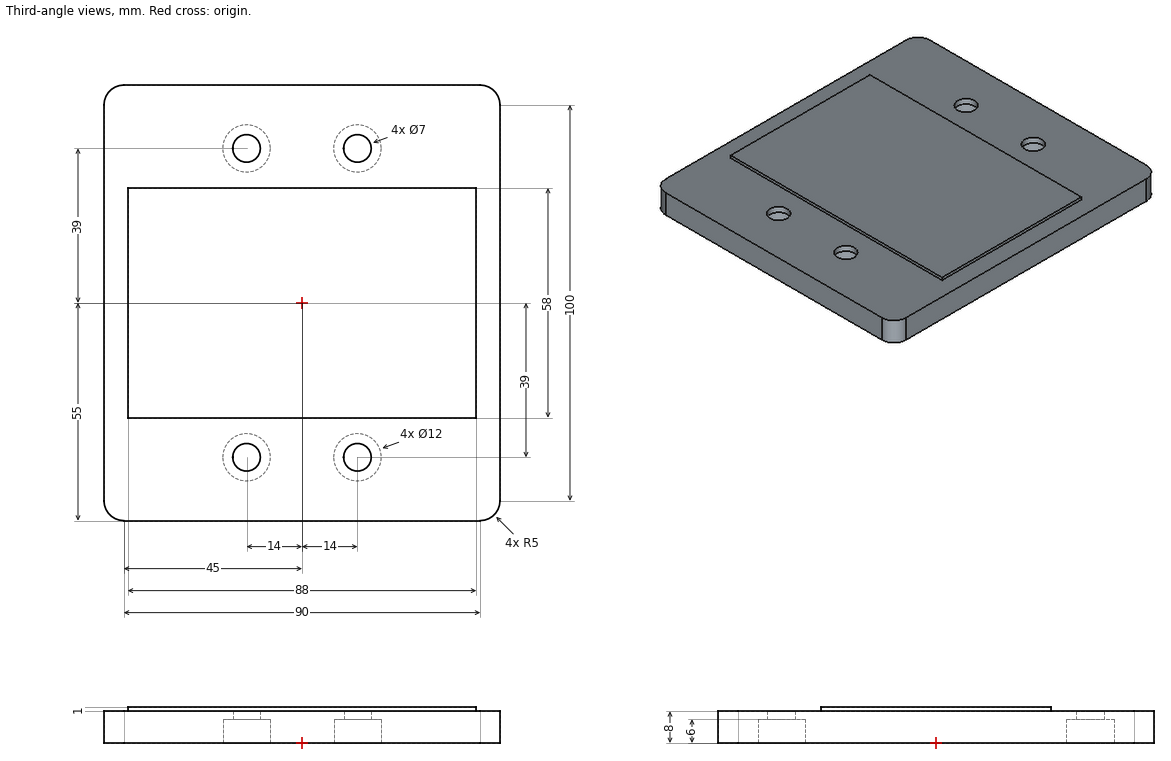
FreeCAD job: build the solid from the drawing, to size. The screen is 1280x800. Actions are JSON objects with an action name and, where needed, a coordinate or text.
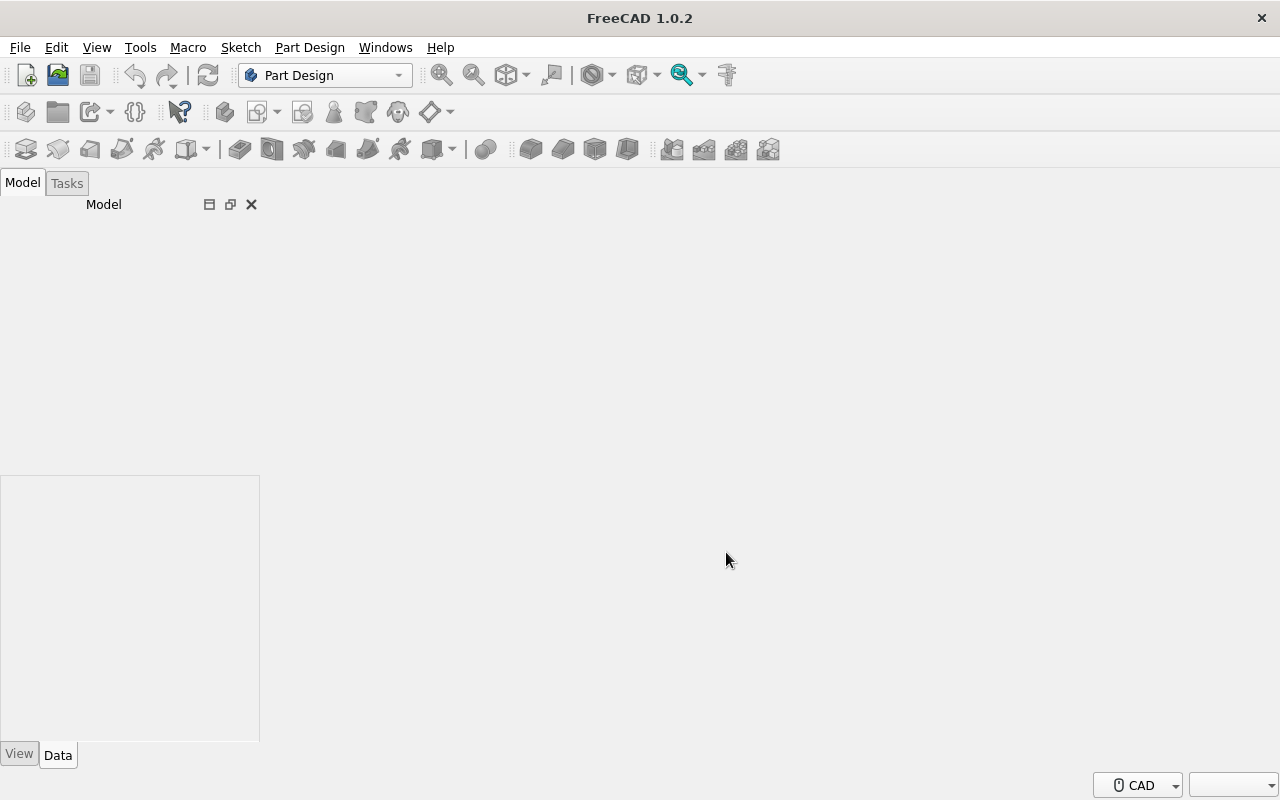
{"action": "key", "text": "ctrl+n"}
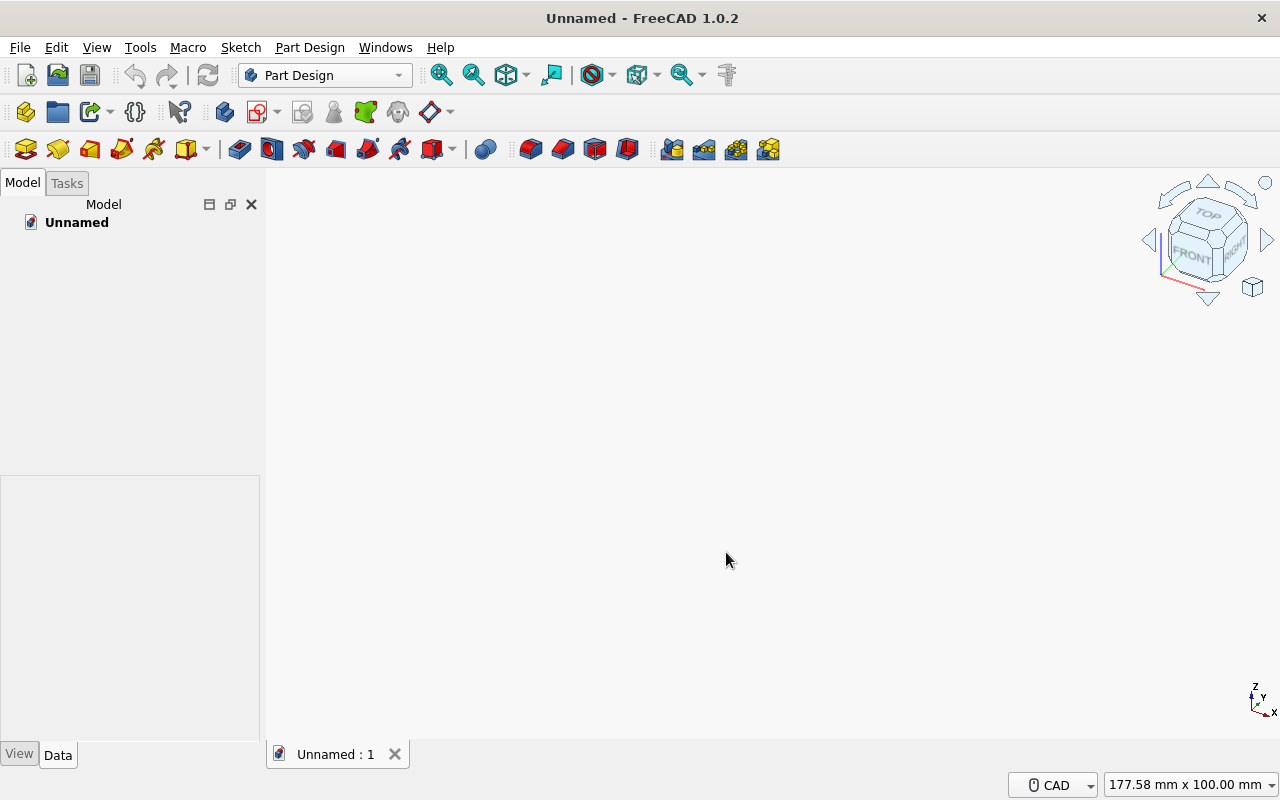
{"action": "left_click", "coordinate": [258, 112]}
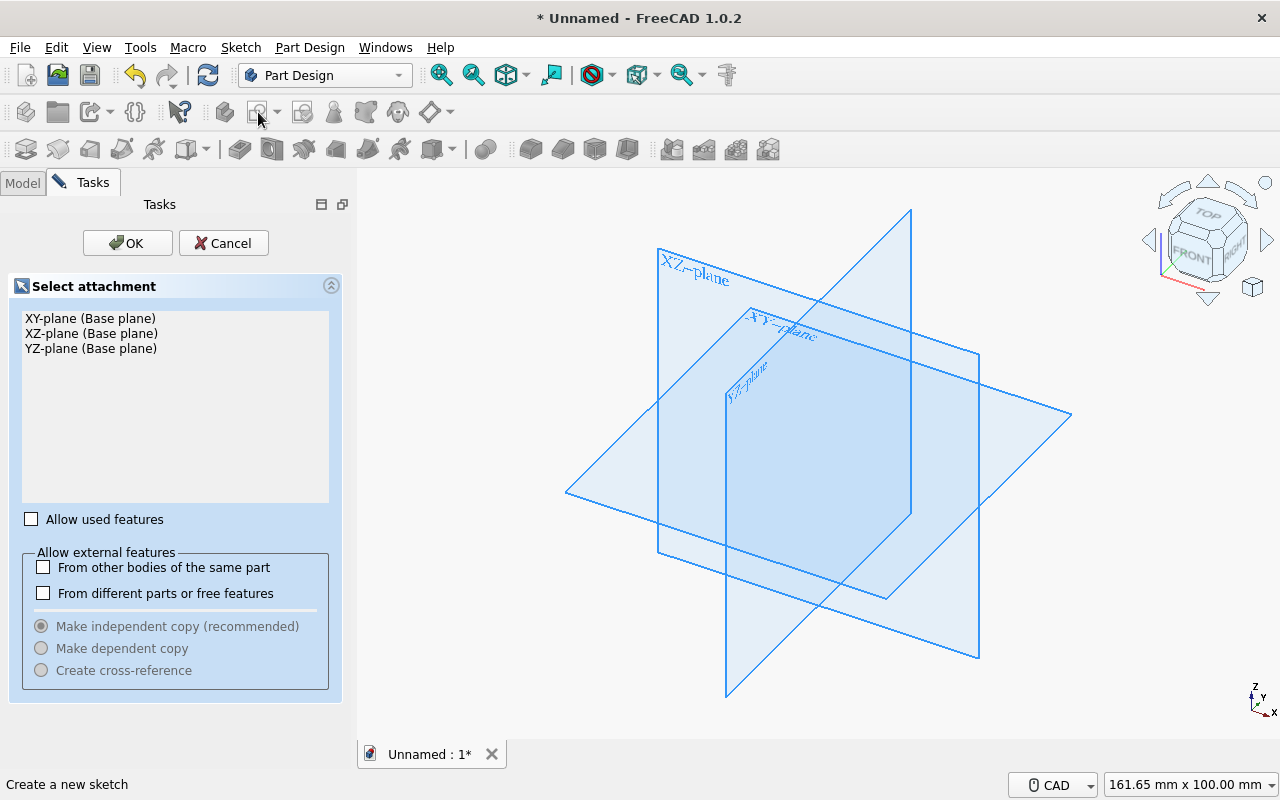
{"action": "left_click", "coordinate": [82, 318]}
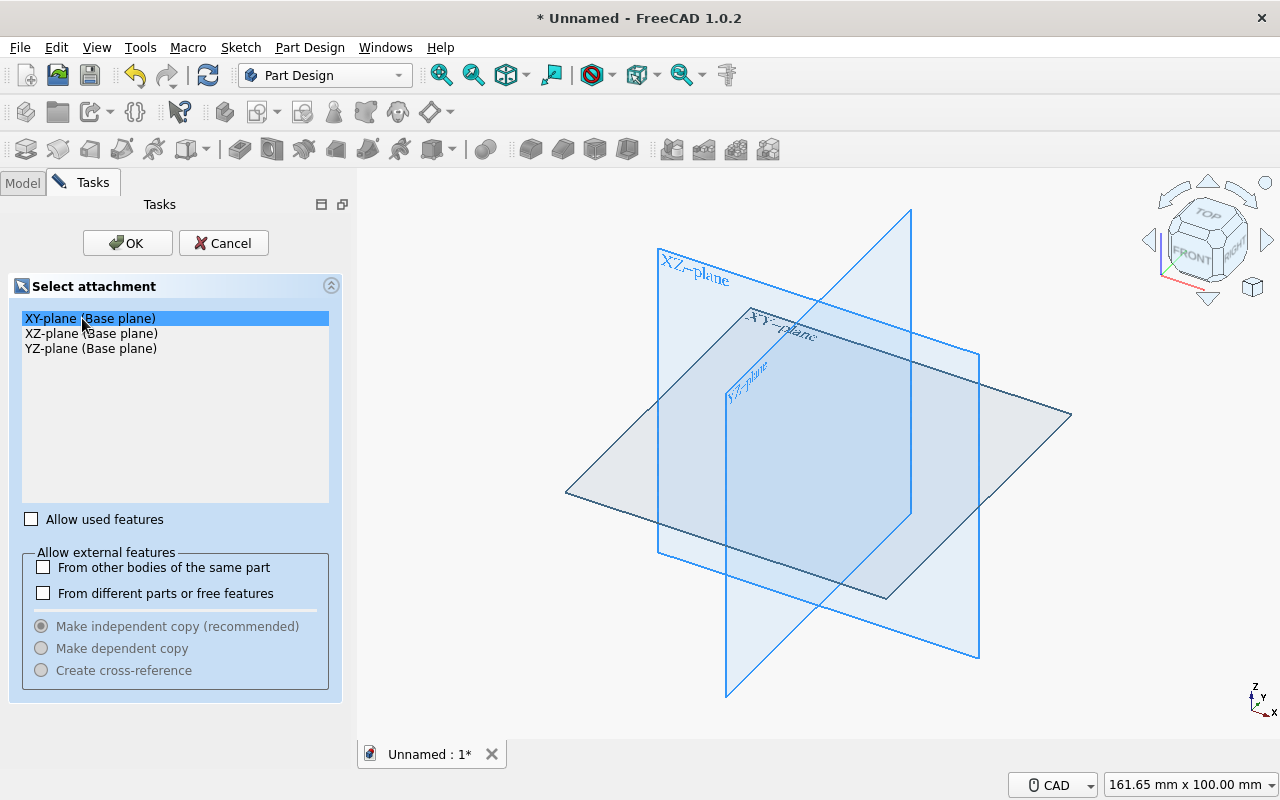
{"action": "left_click", "coordinate": [128, 243]}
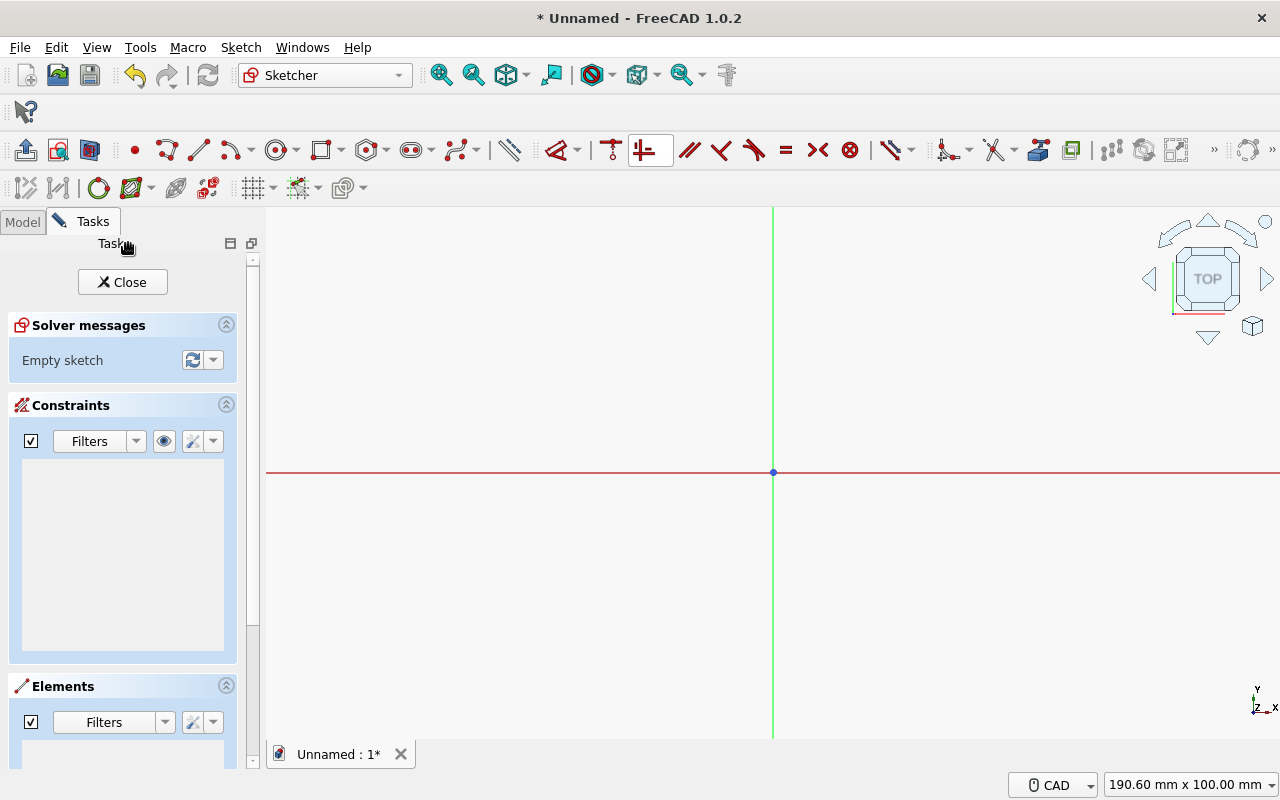
{"action": "scroll", "coordinate": [621, 473], "scroll_direction": "down", "scroll_amount": 3}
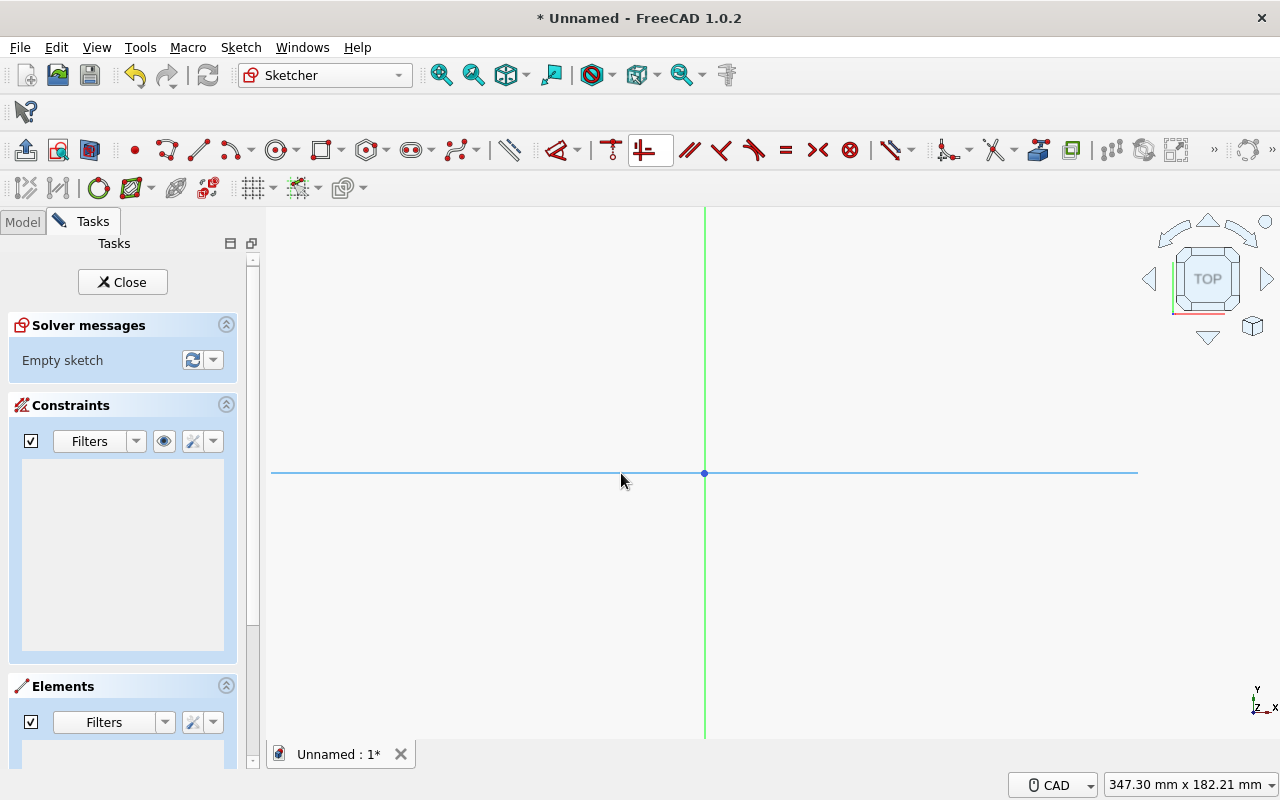
{"action": "key", "text": "g l"}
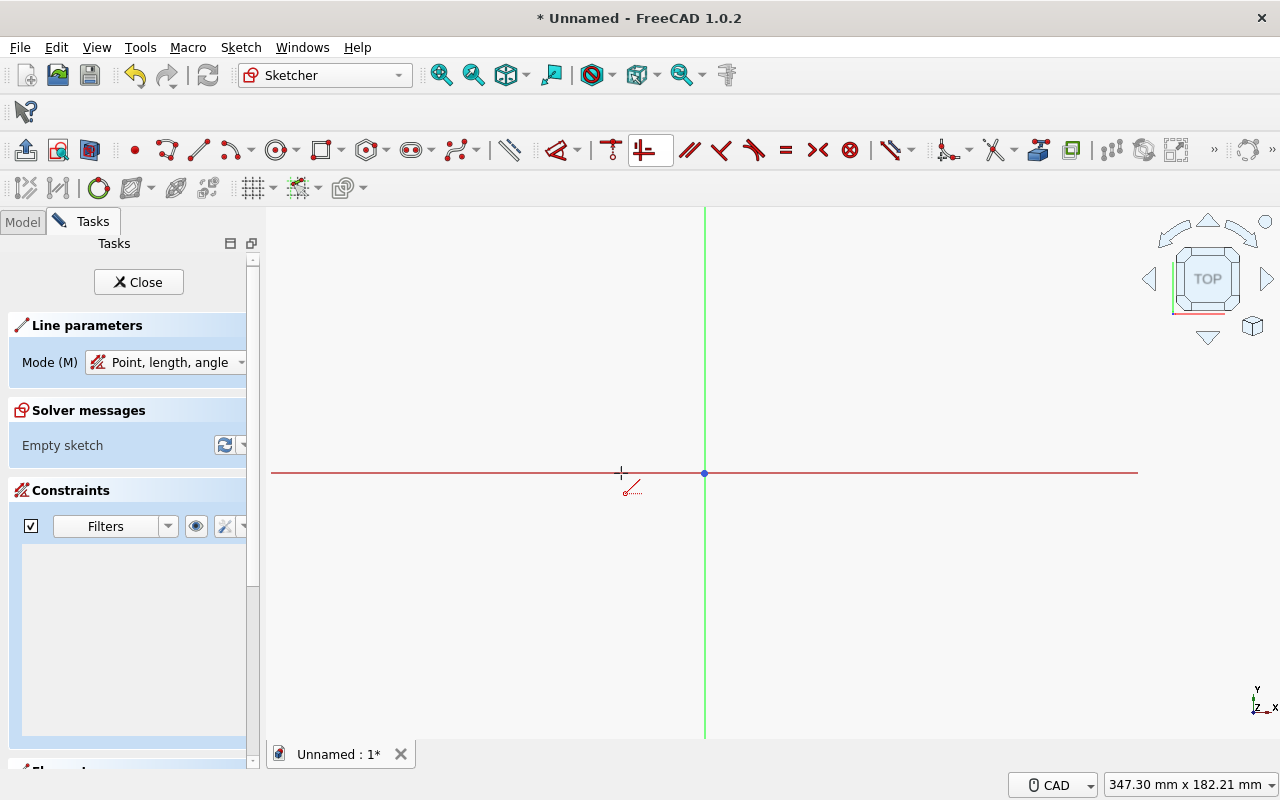
{"action": "left_click", "coordinate": [573, 634]}
{"action": "left_click", "coordinate": [836, 634]}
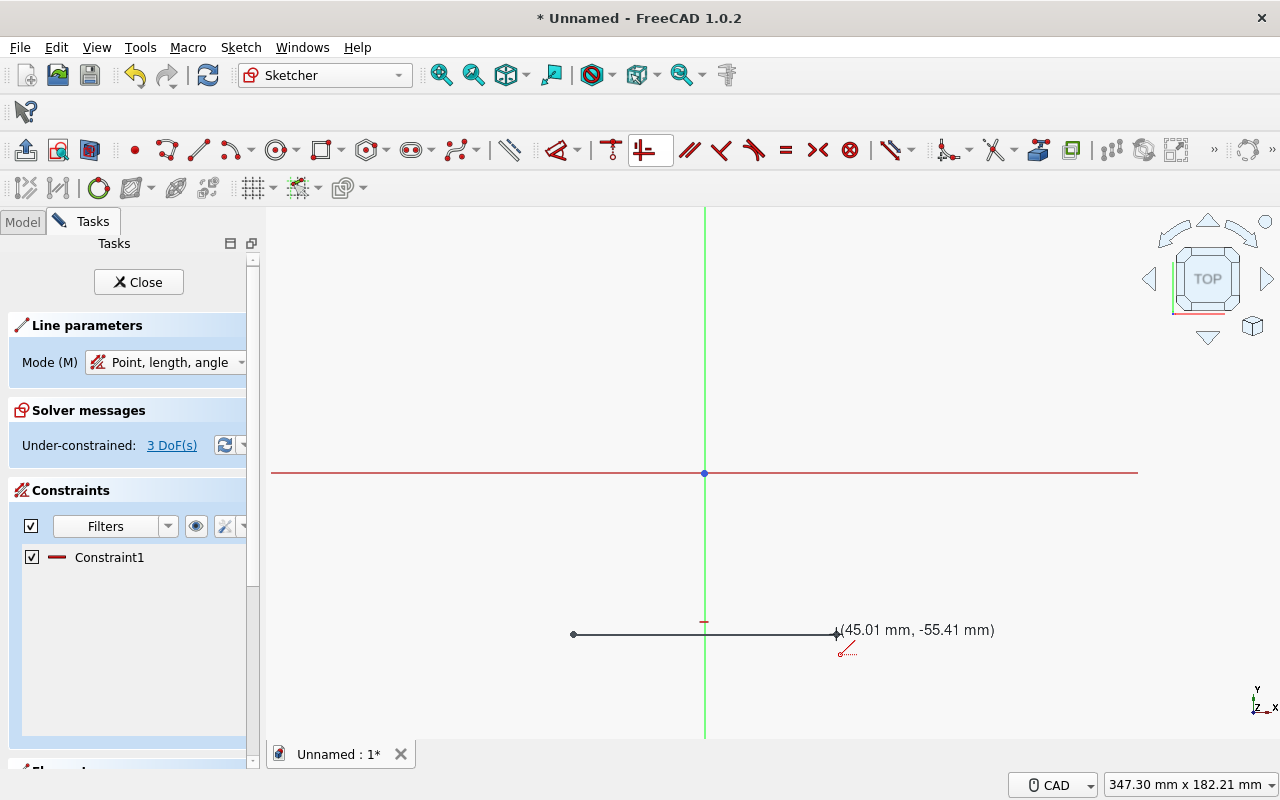
{"action": "left_click", "coordinate": [851, 619]}
{"action": "left_click", "coordinate": [851, 327]}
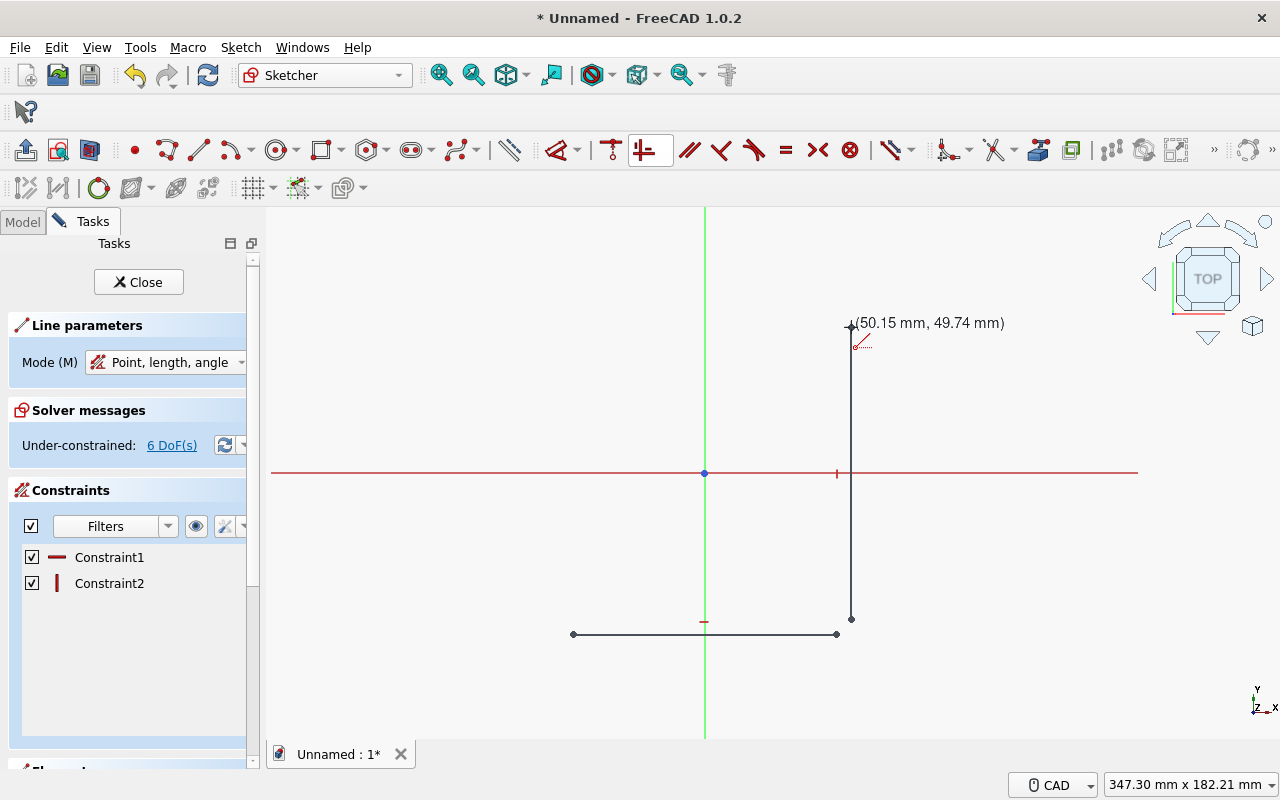
{"action": "left_click", "coordinate": [836, 313]}
{"action": "left_click", "coordinate": [573, 313]}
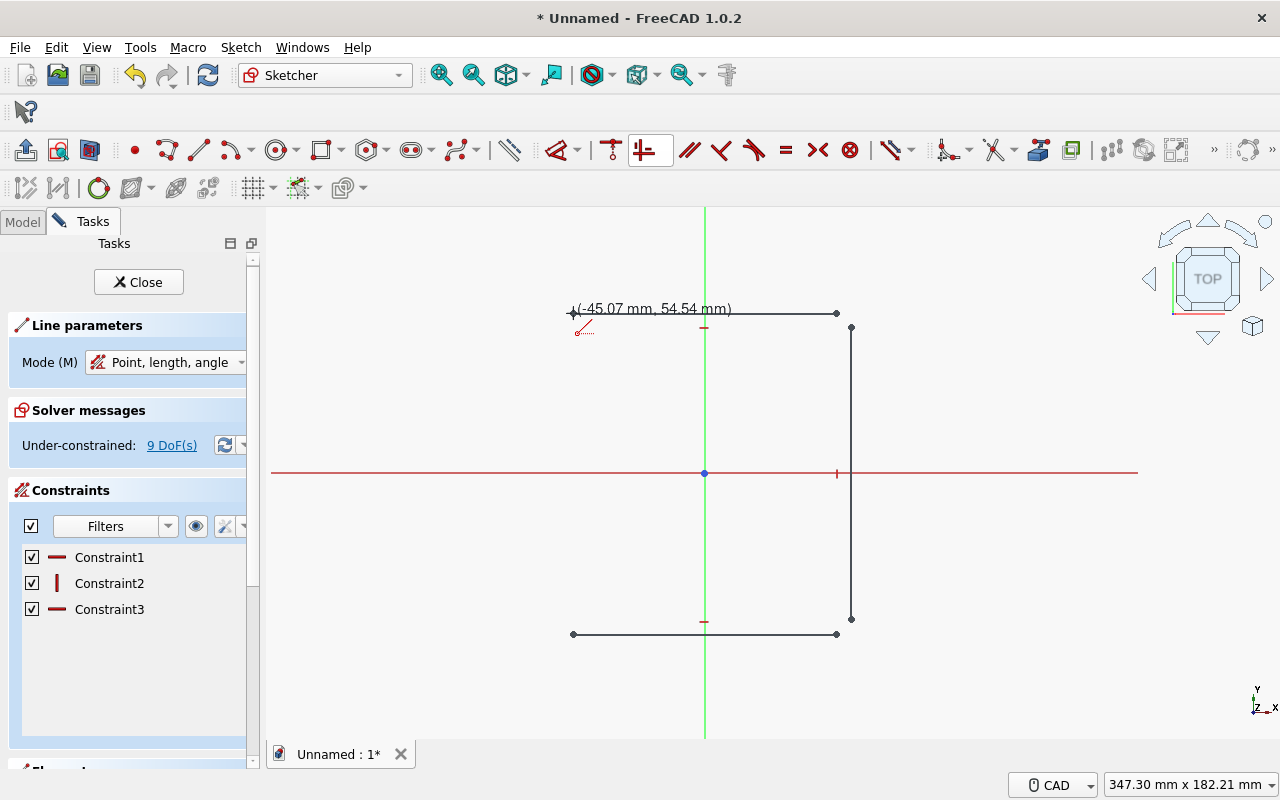
{"action": "left_click", "coordinate": [559, 327]}
{"action": "left_click", "coordinate": [559, 619]}